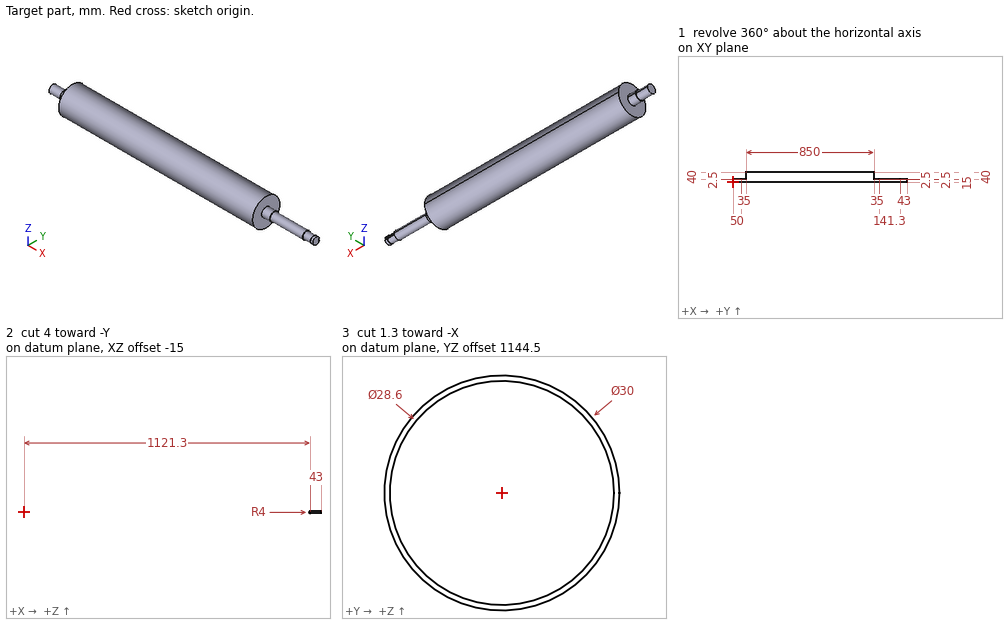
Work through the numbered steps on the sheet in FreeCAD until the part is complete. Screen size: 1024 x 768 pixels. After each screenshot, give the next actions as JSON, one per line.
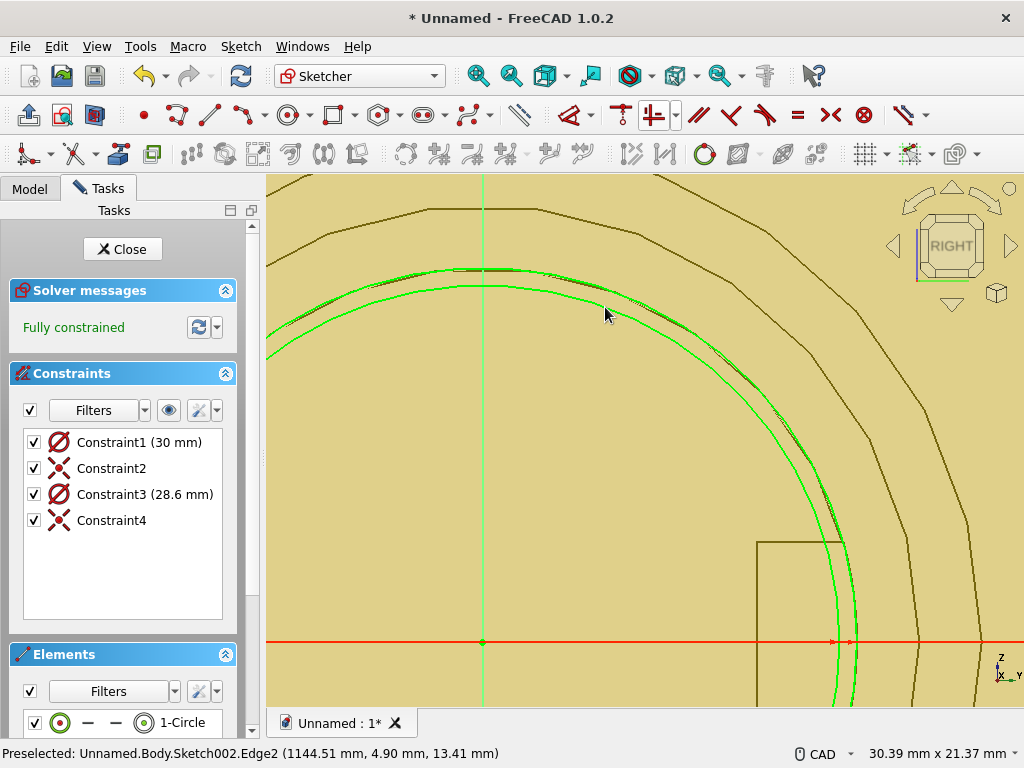
{"action": "left_click", "coordinate": [123, 249]}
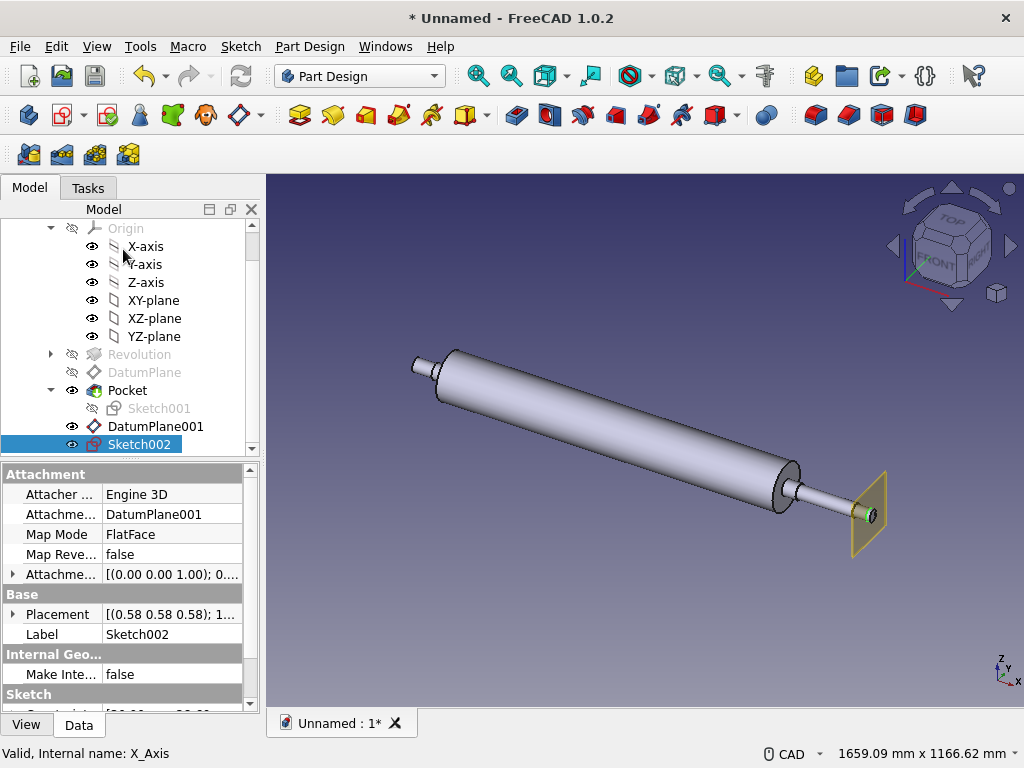
{"action": "left_click", "coordinate": [517, 116]}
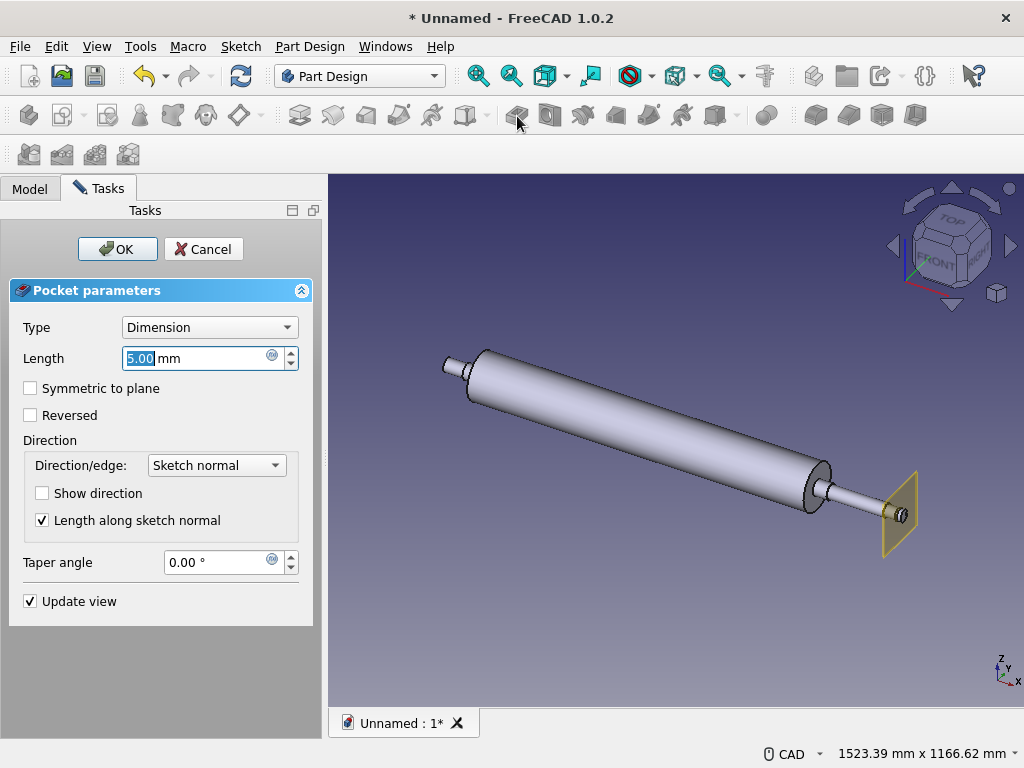
{"action": "type", "text": "1.3"}
{"action": "key", "text": "Tab"}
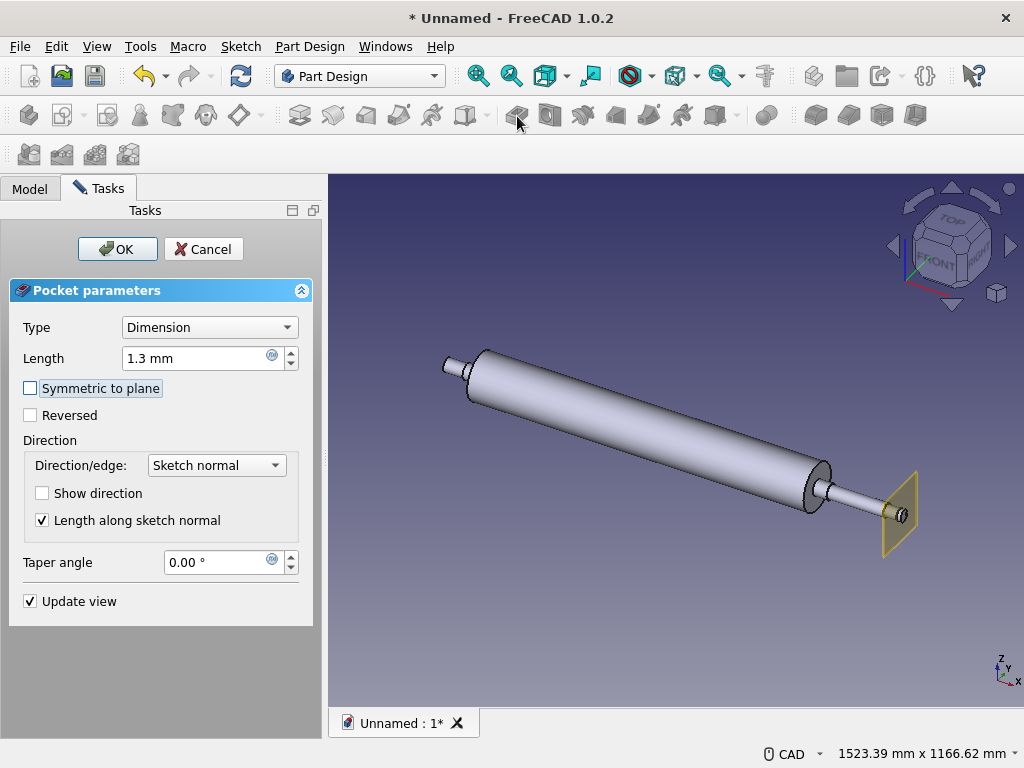
{"action": "left_click", "coordinate": [118, 249]}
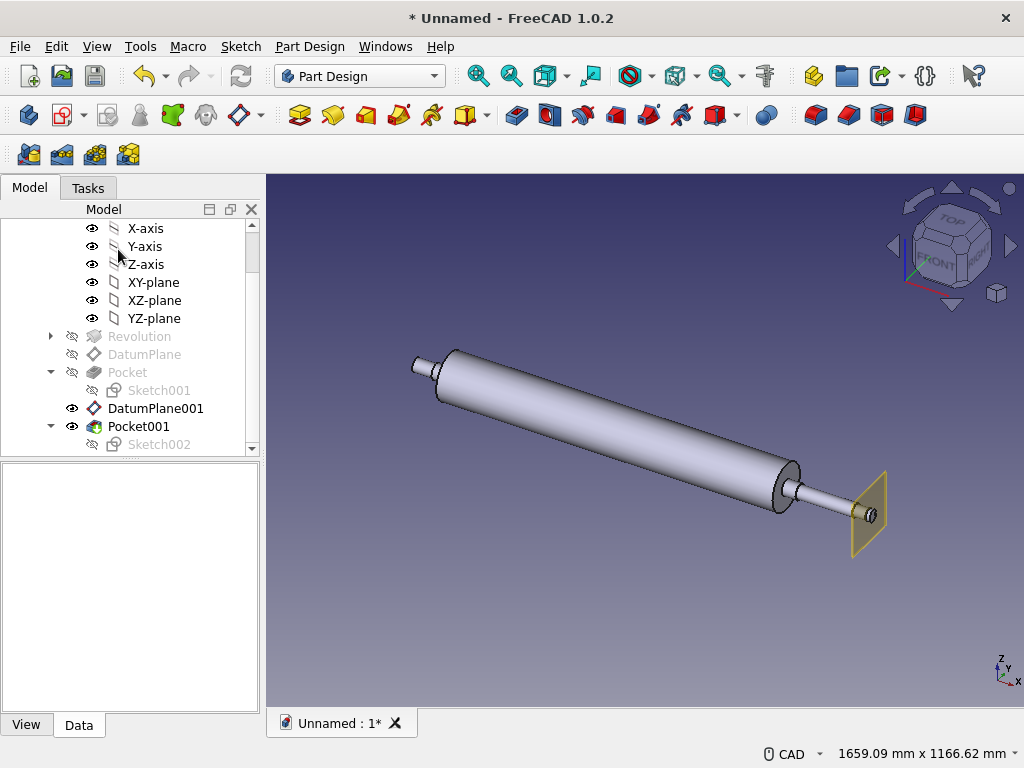
{"action": "left_click", "coordinate": [117, 408]}
{"action": "key", "text": "space"}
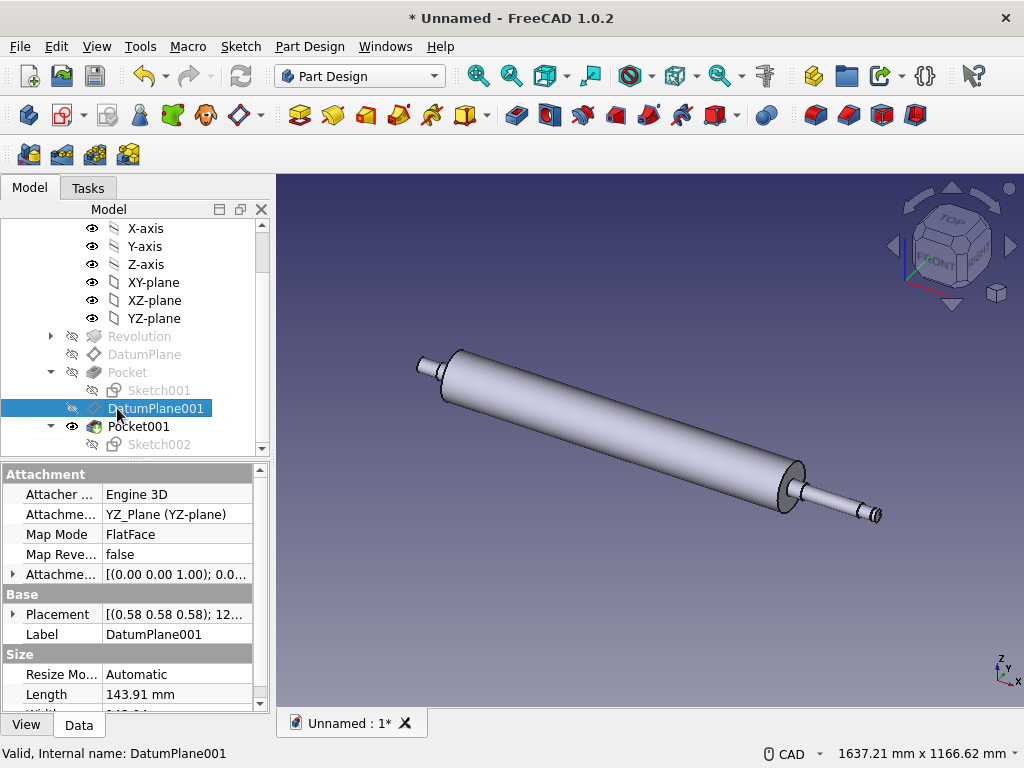
{"action": "key", "text": "0"}